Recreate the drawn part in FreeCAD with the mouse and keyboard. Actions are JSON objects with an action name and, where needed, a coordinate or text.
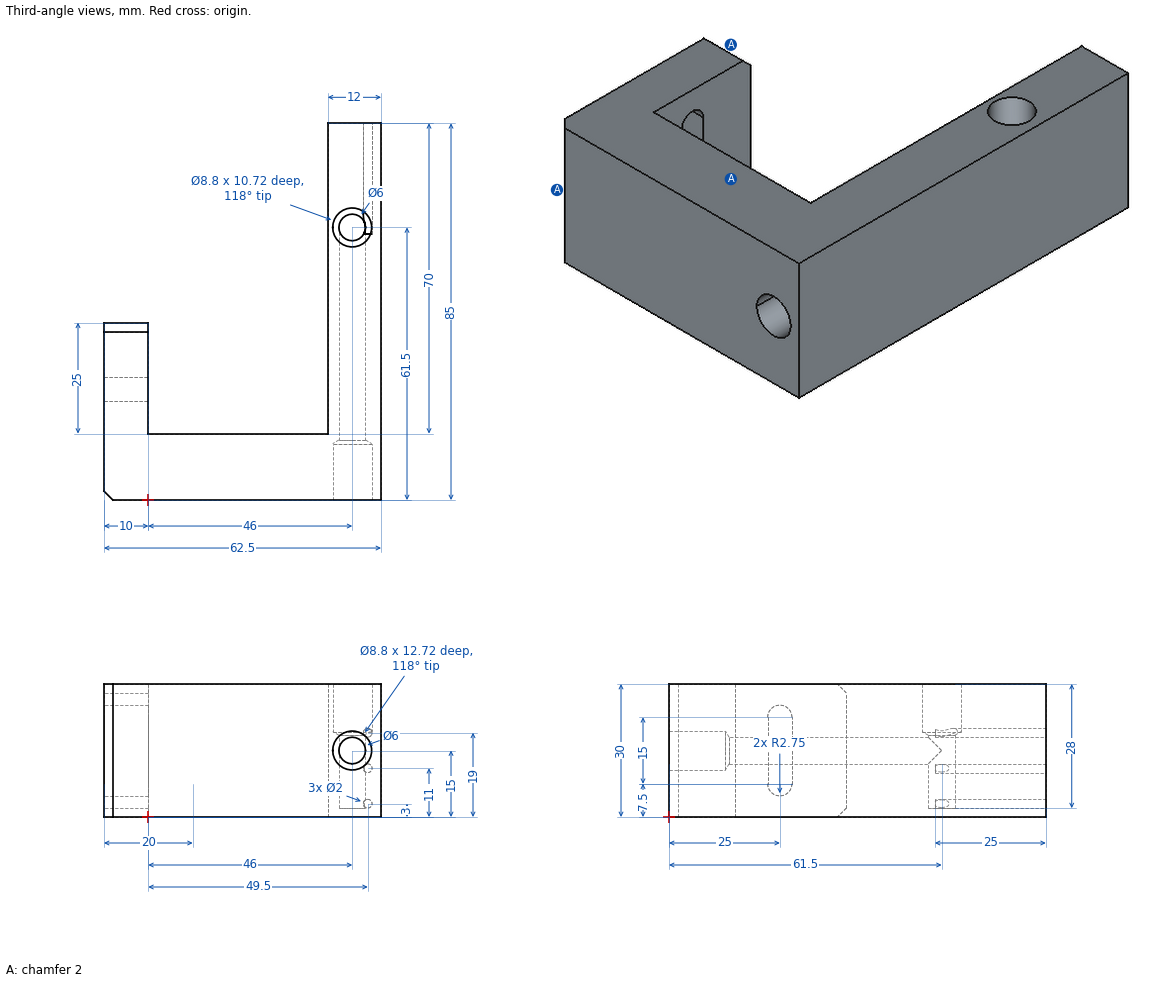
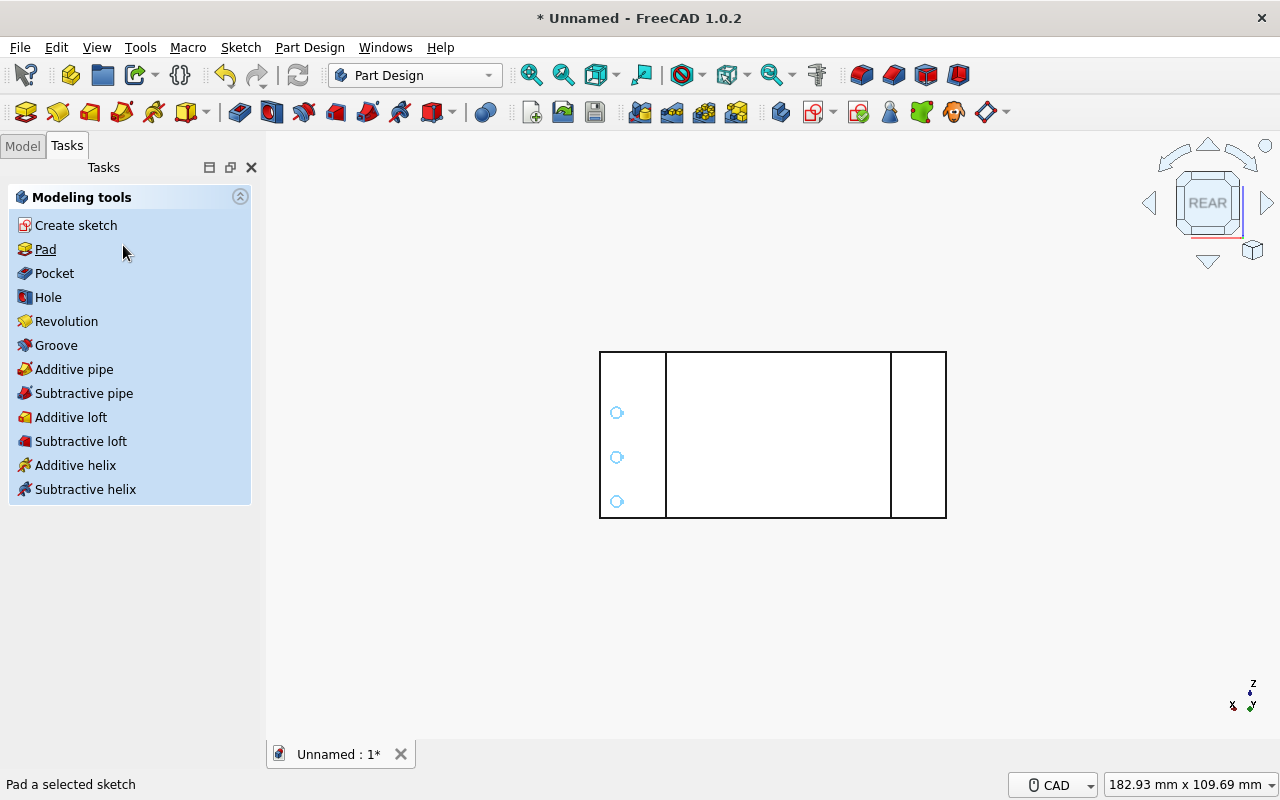
{"action": "left_click", "coordinate": [240, 112]}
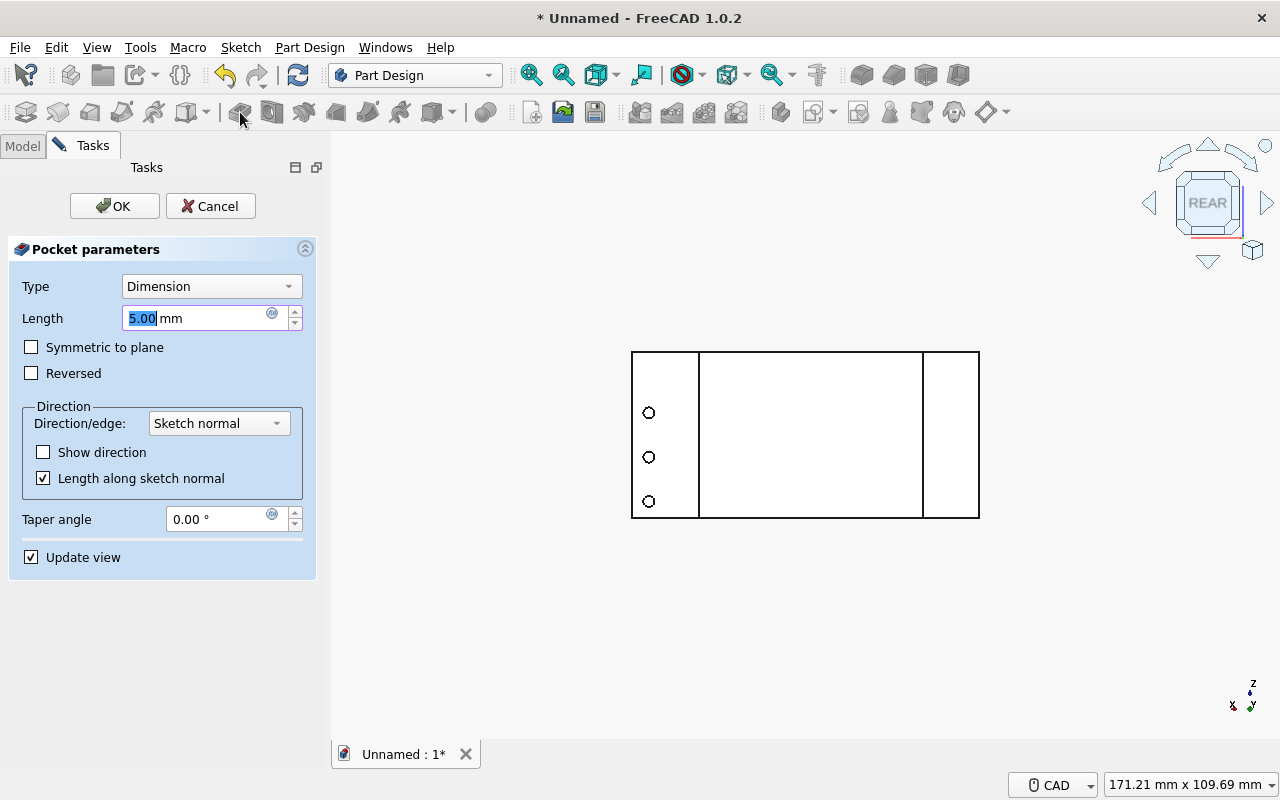
{"action": "type", "text": "25"}
{"action": "key", "text": "Tab"}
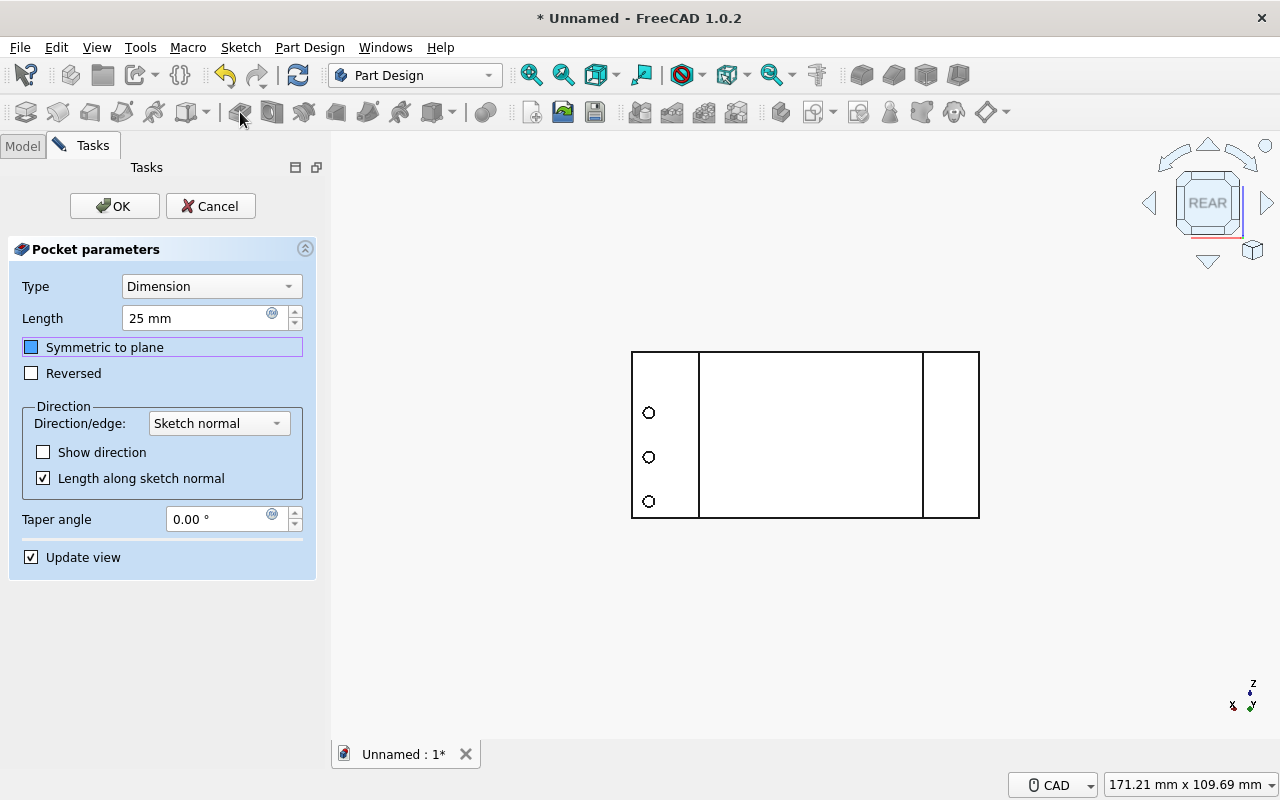
{"action": "left_click", "coordinate": [115, 206]}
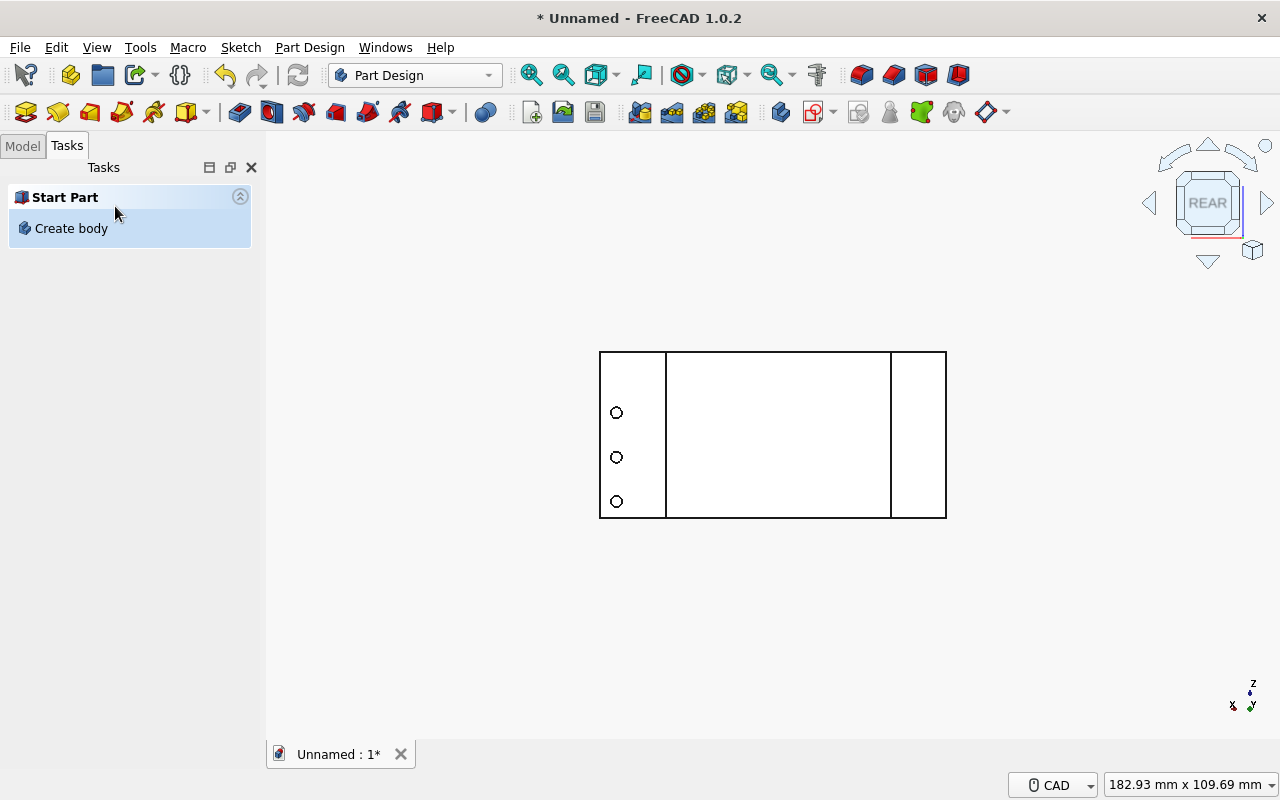
{"action": "key", "text": "v f"}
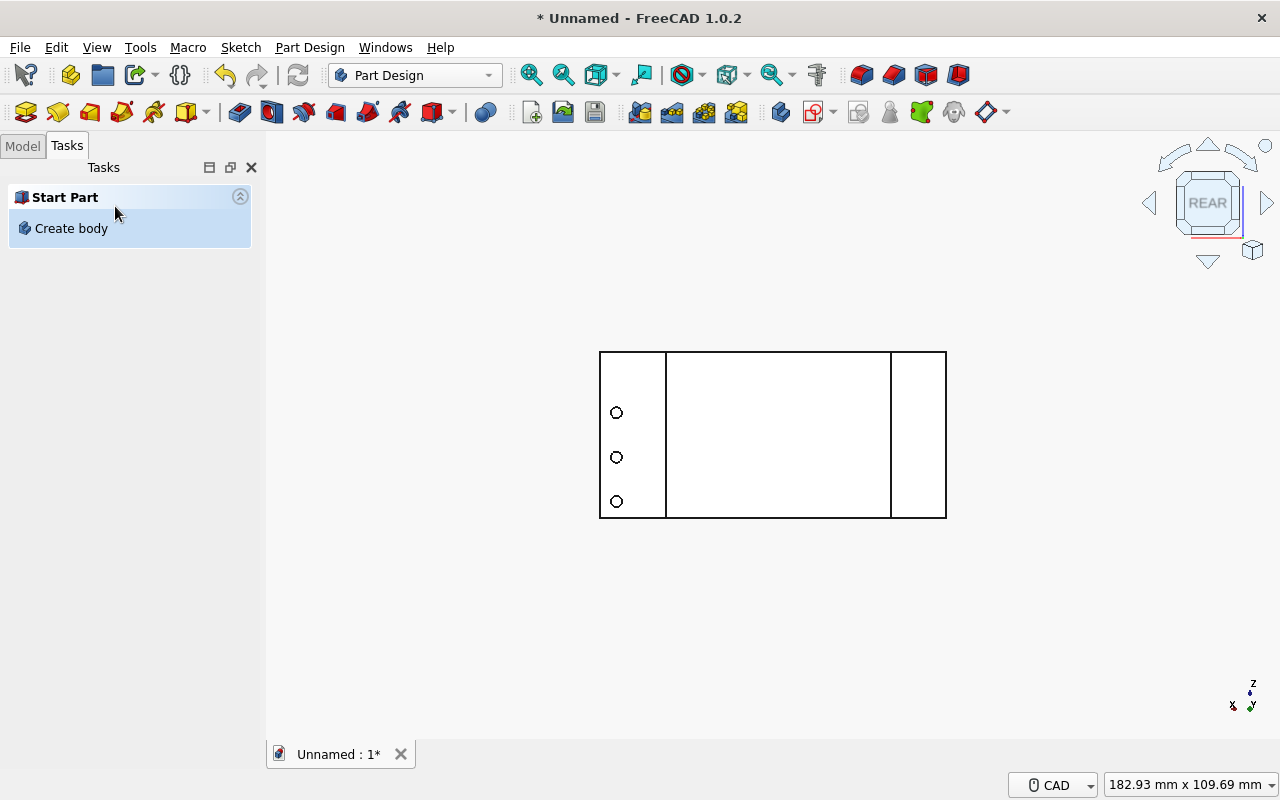
{"action": "key", "text": "0"}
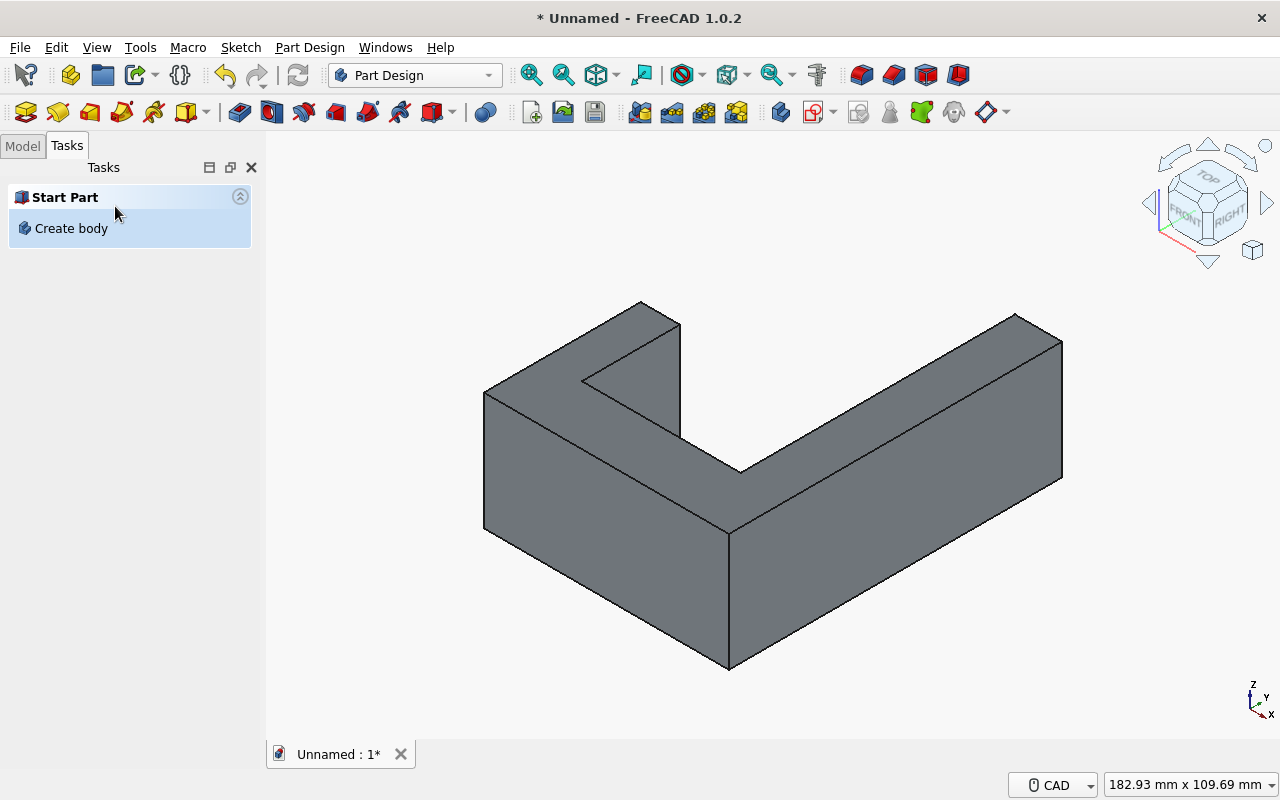
{"action": "left_click", "coordinate": [700, 489]}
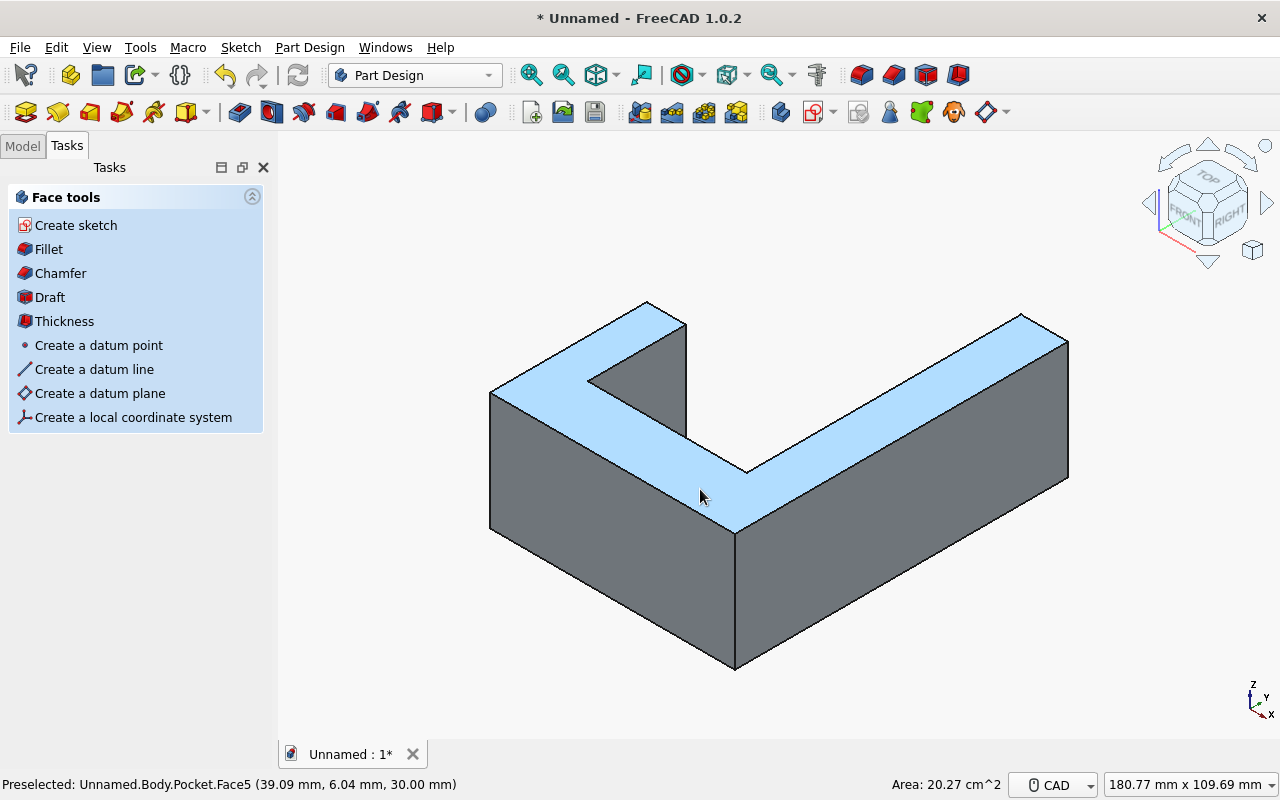
{"action": "left_click", "coordinate": [814, 112]}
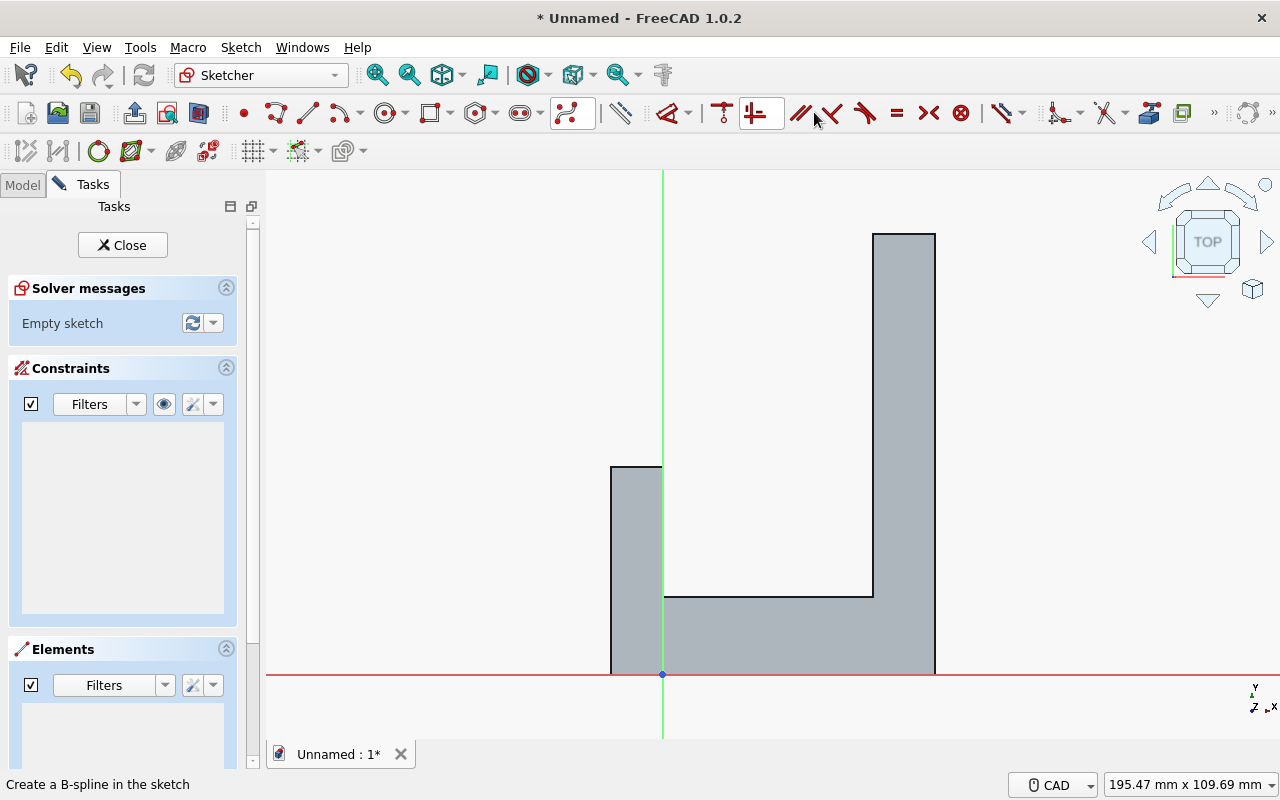
{"action": "scroll", "coordinate": [921, 346], "scroll_direction": "up", "scroll_amount": 12}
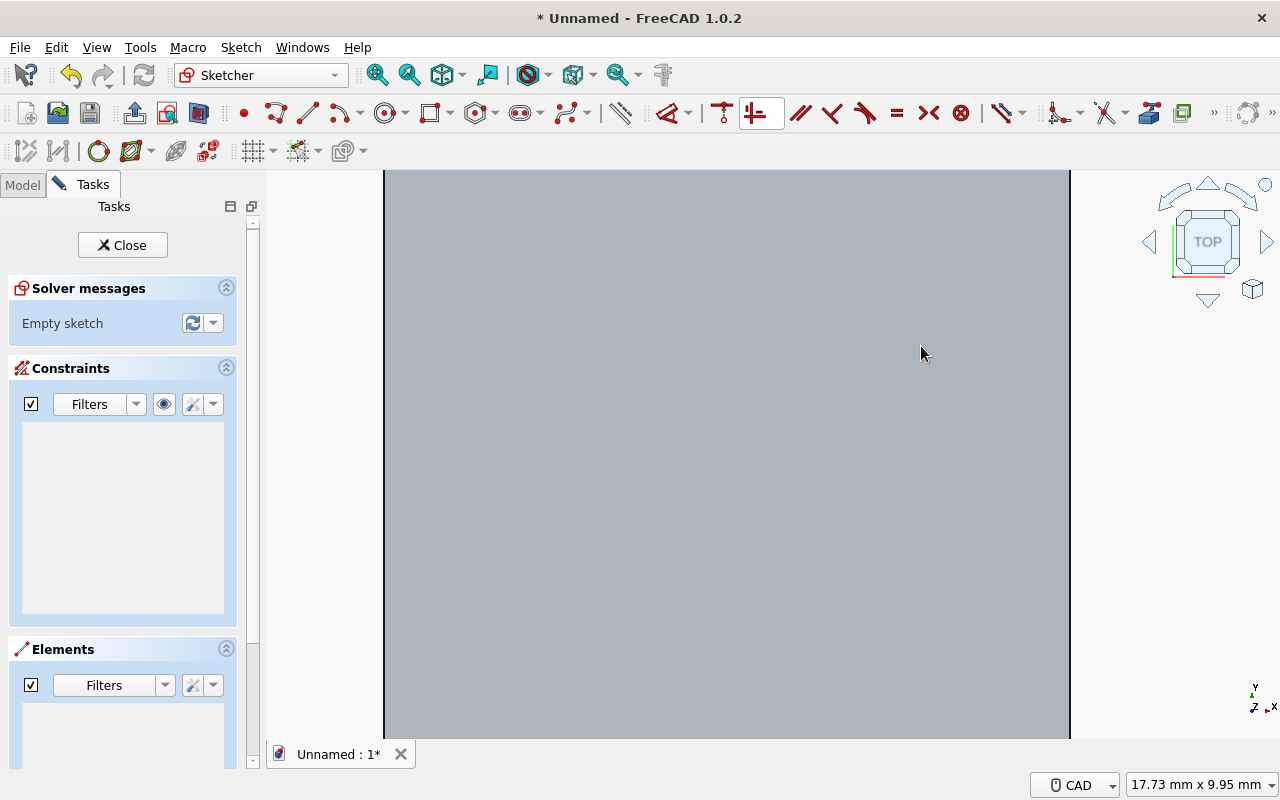
{"action": "key", "text": "g c"}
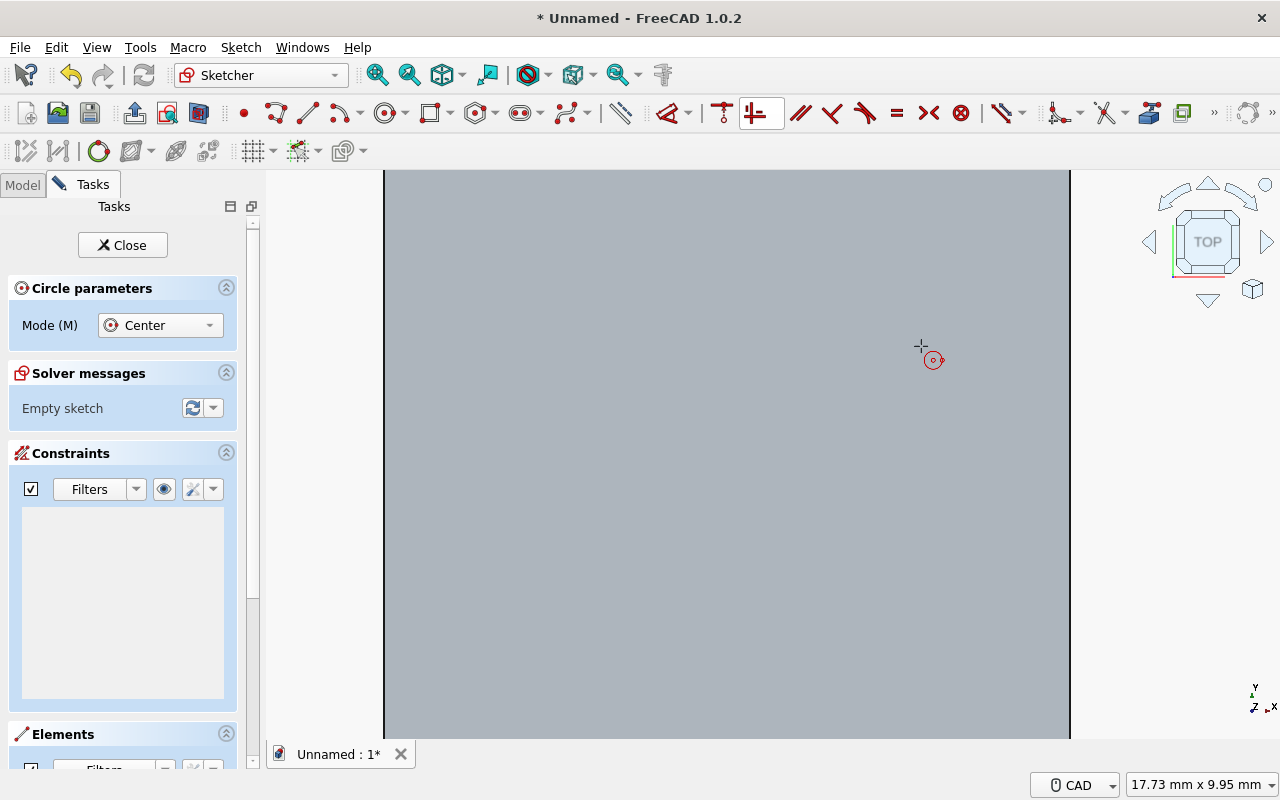
{"action": "left_click", "coordinate": [698, 452]}
{"action": "mouse_move", "coordinate": [820, 331]}